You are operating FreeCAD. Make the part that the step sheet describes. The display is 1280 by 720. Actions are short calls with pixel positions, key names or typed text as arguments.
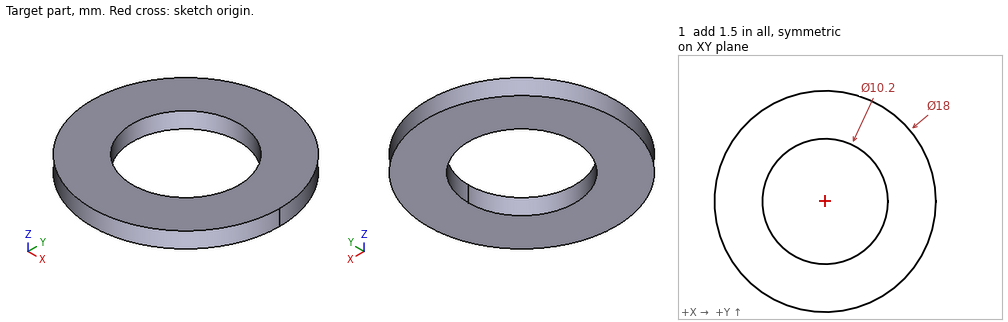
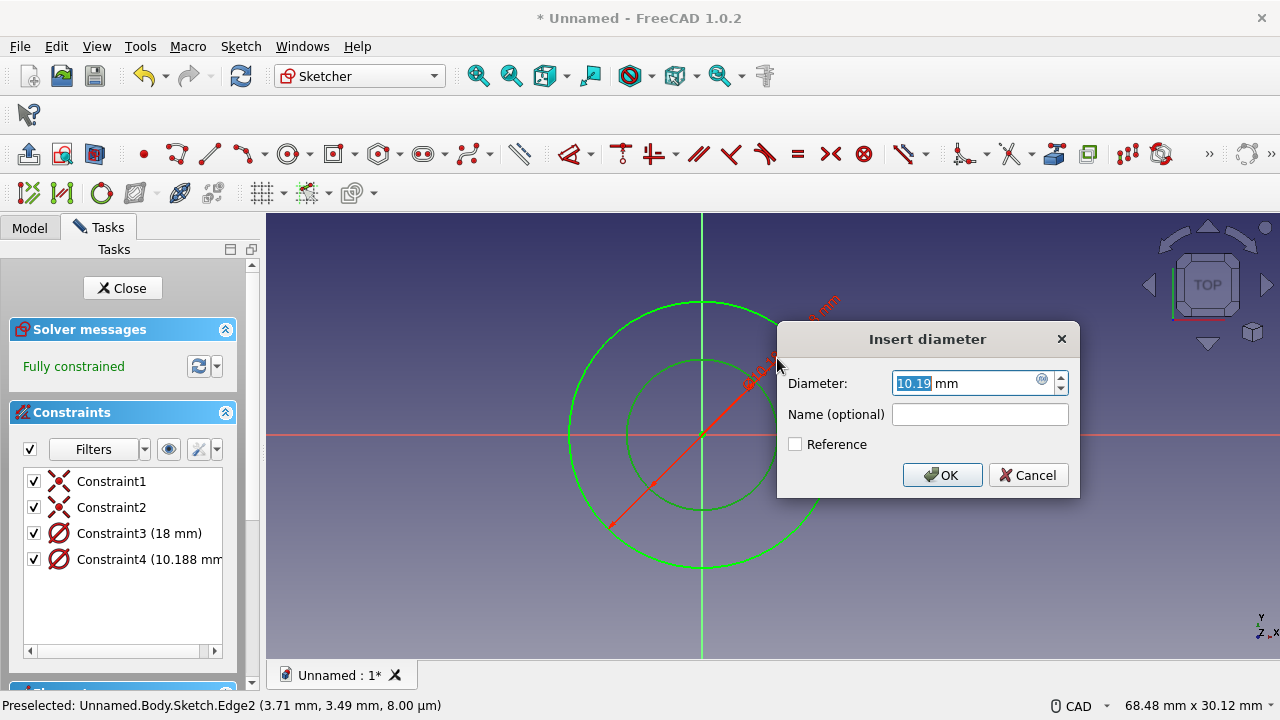
text(10.2)
key(Return)
key(Escape)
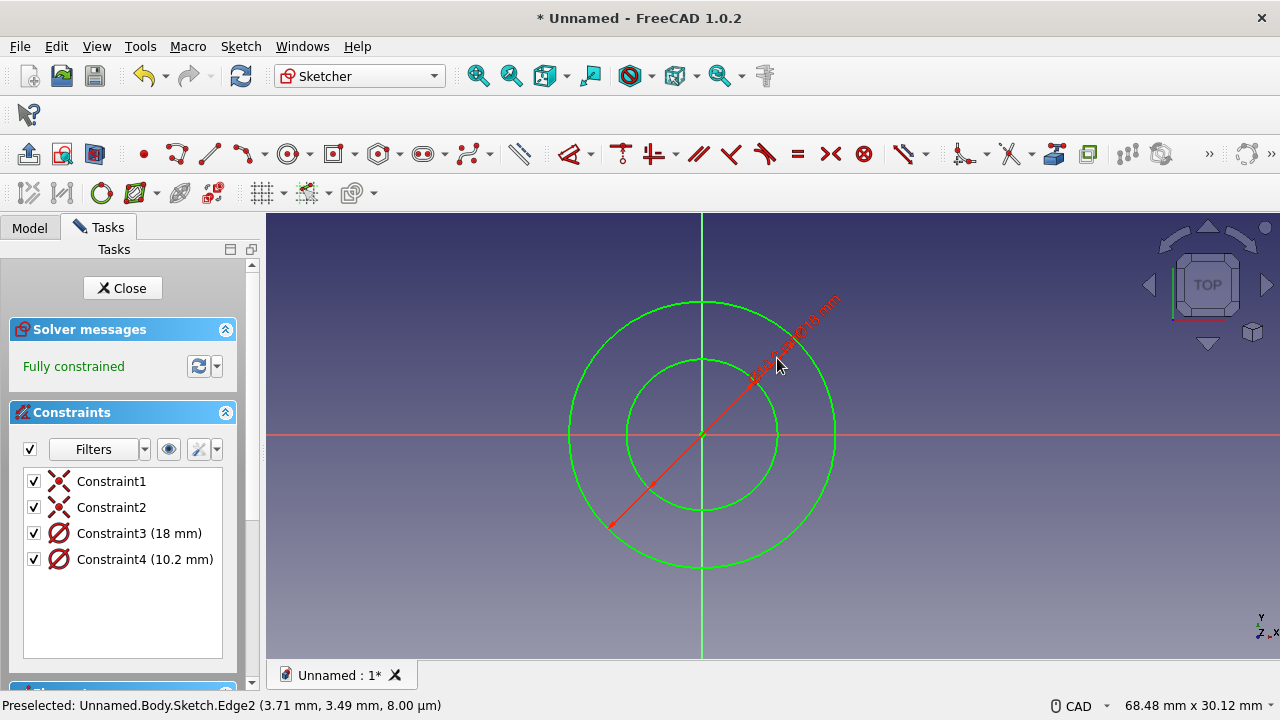
click(123, 288)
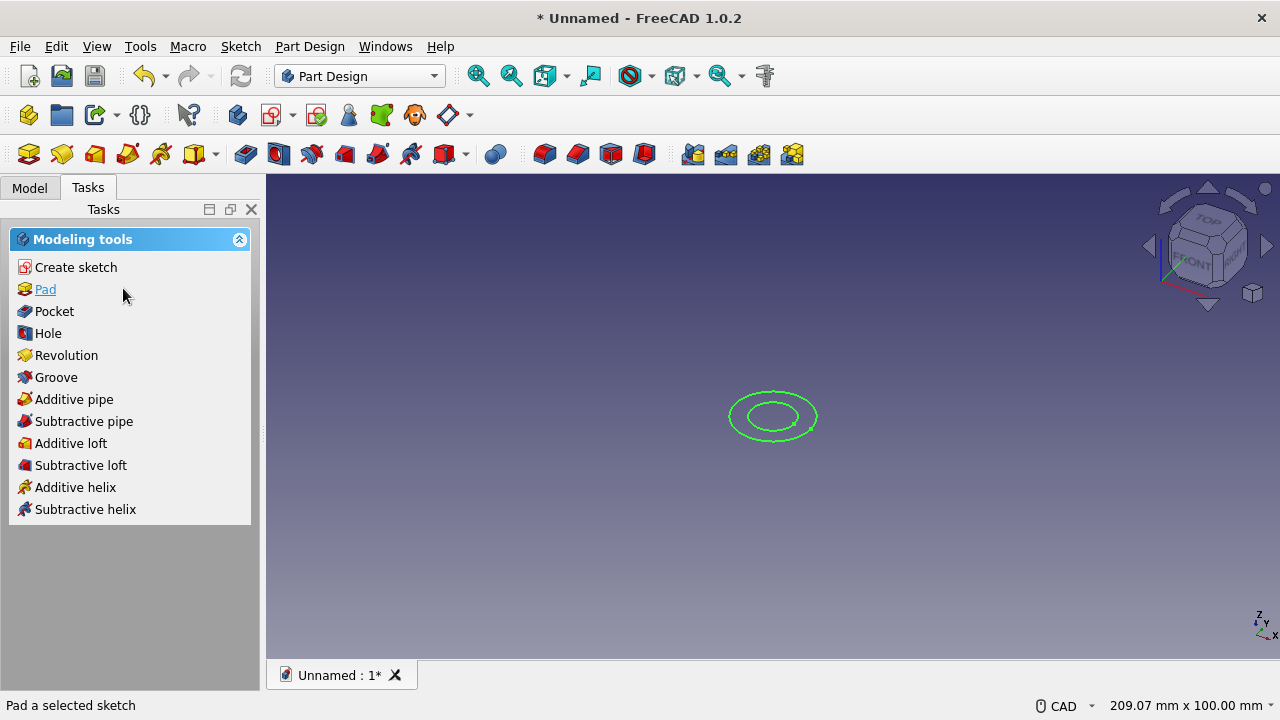
click(29, 154)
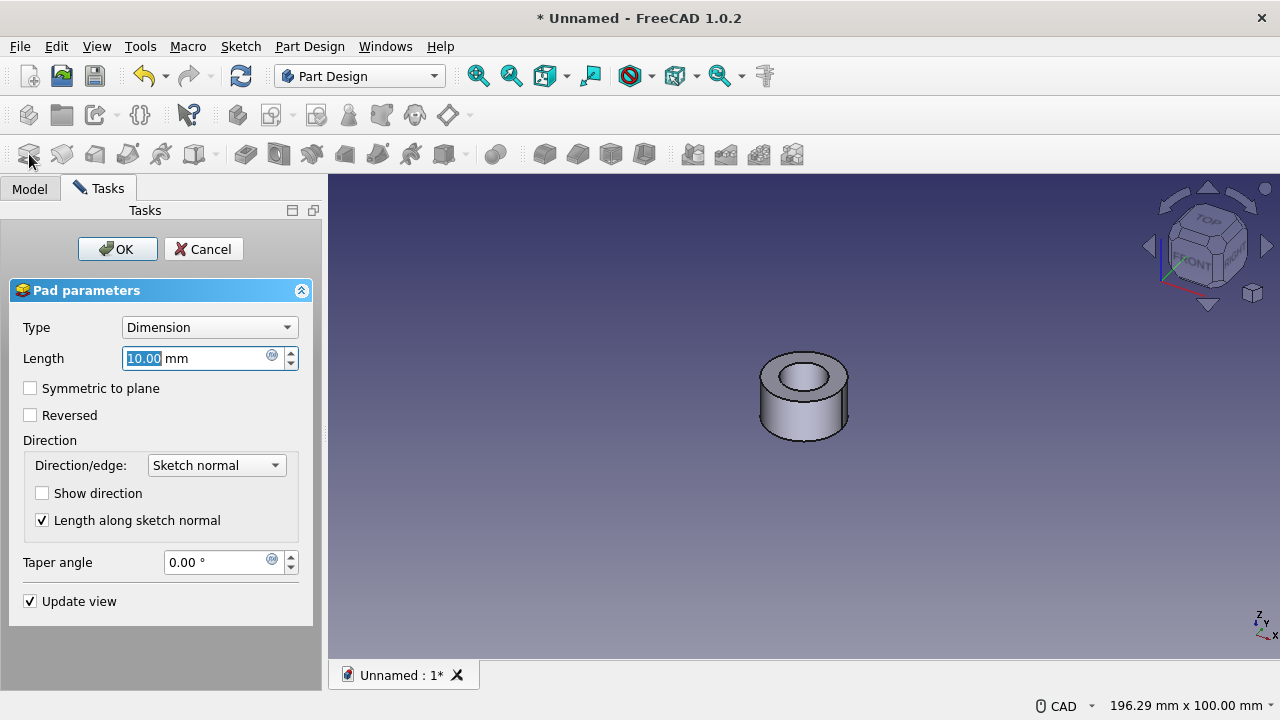
text(1.5)
key(Tab)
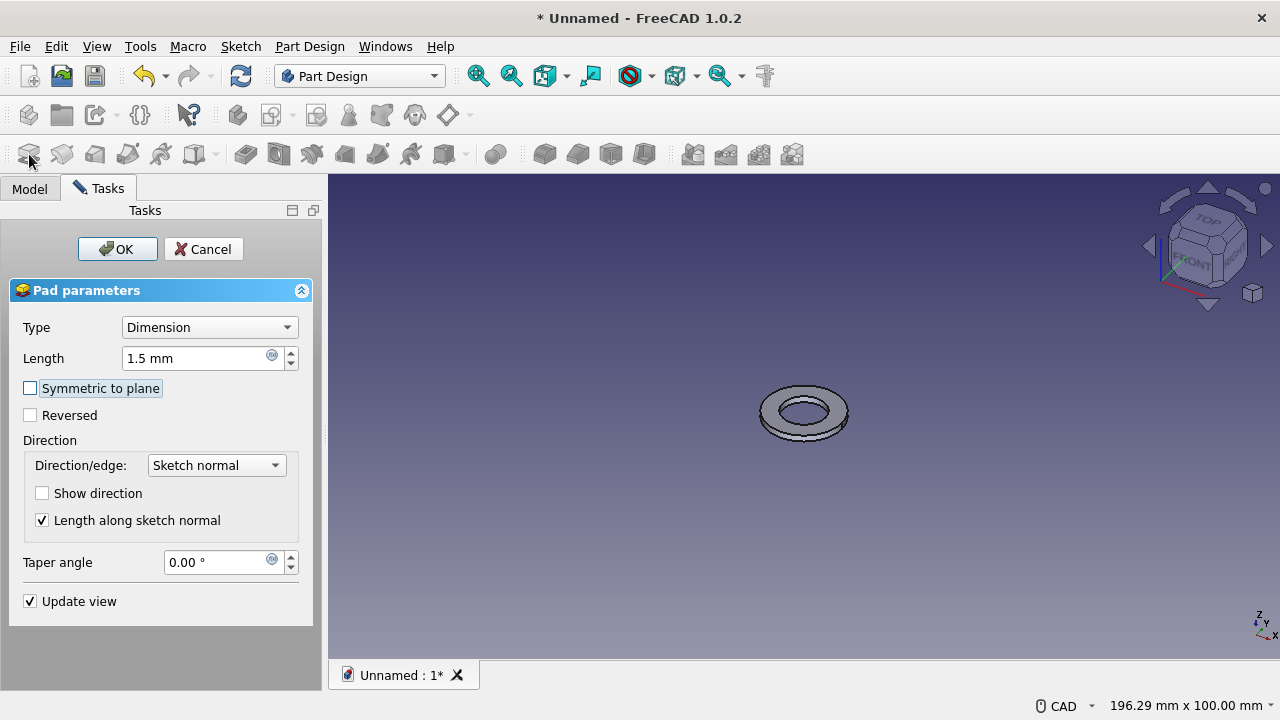
click(31, 388)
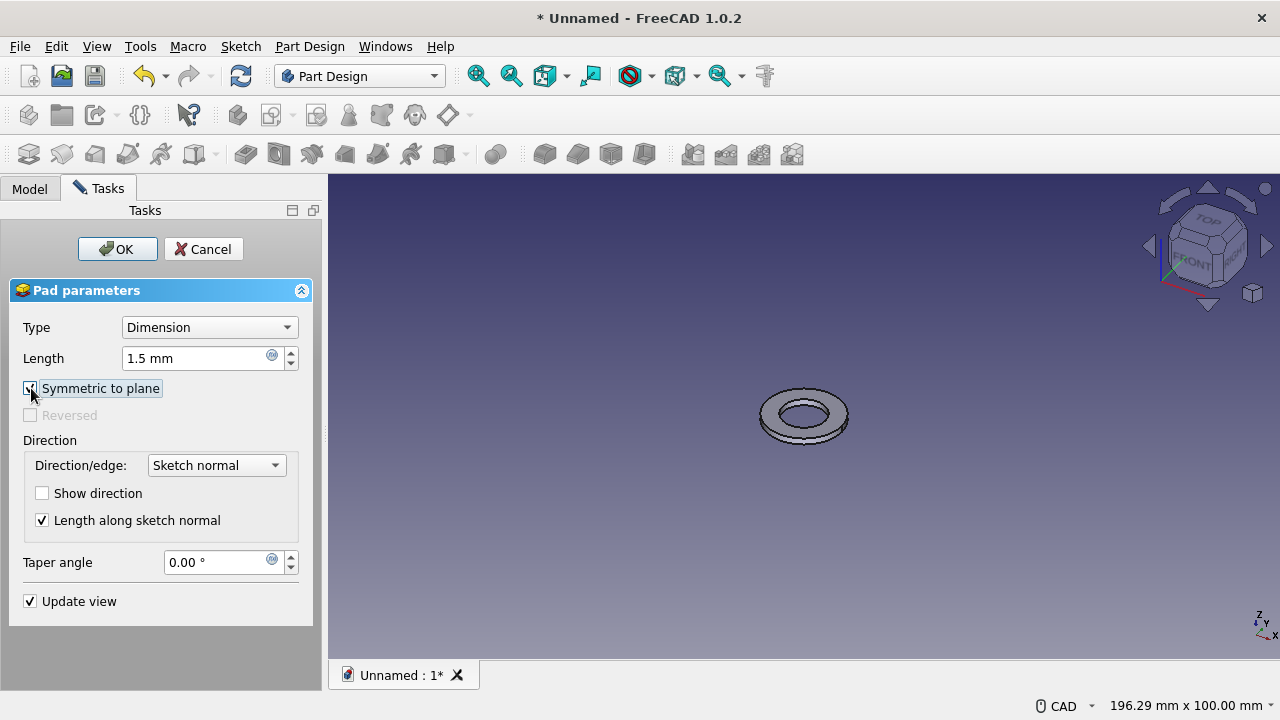
click(118, 249)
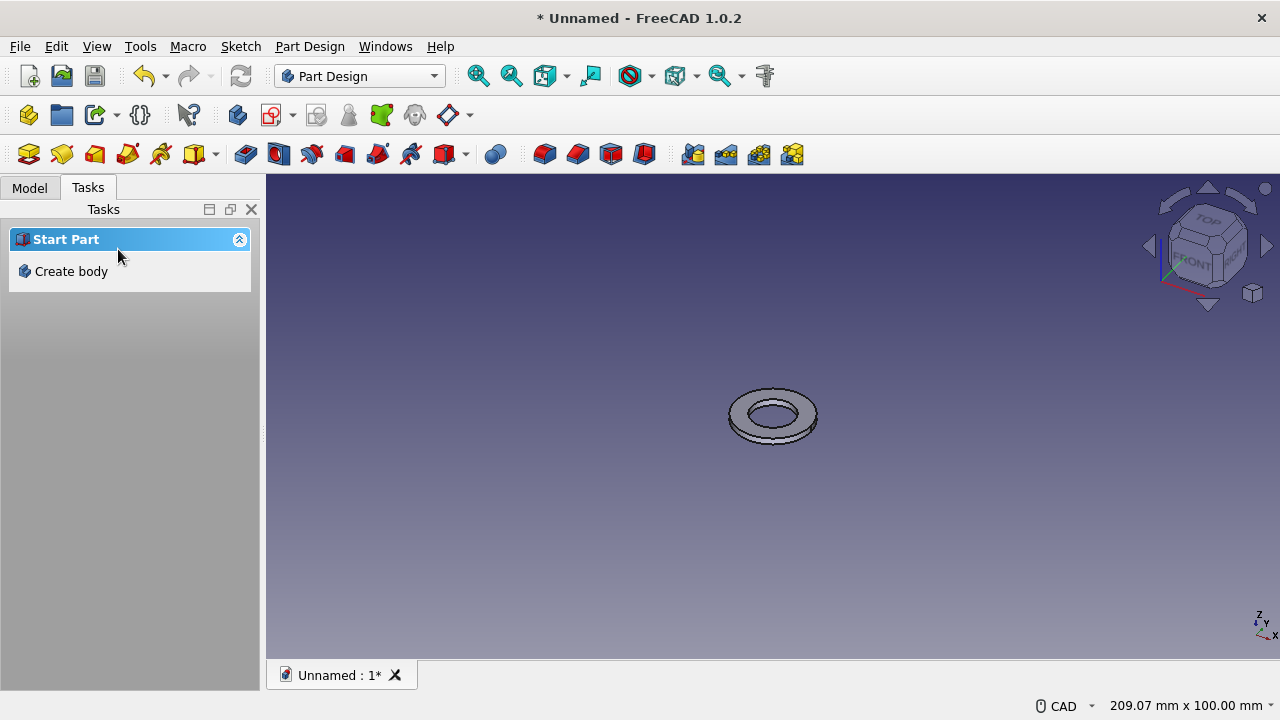
key(0)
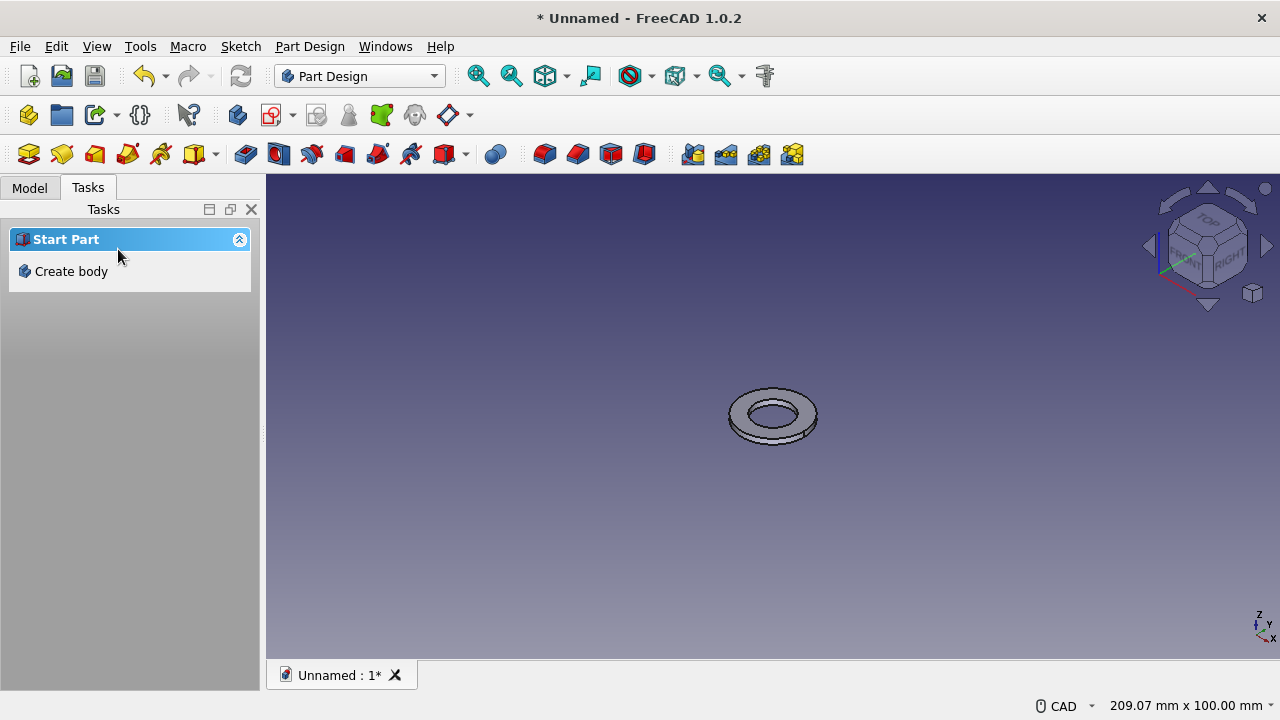
click(479, 76)